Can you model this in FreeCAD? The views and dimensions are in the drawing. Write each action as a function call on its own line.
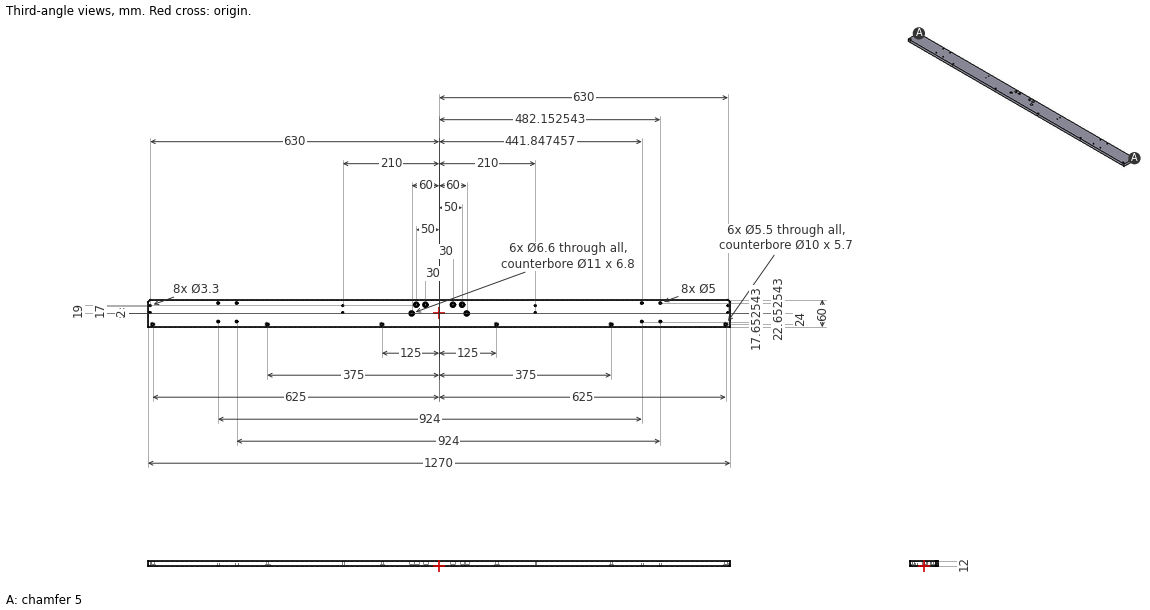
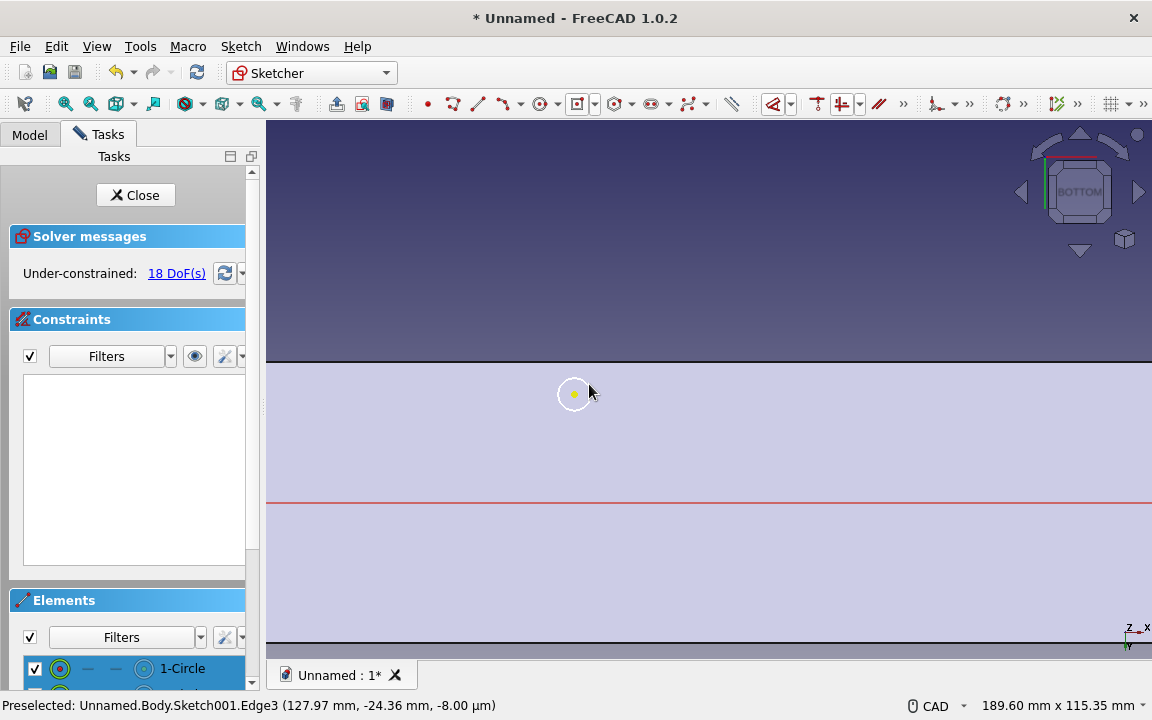
click(586, 383)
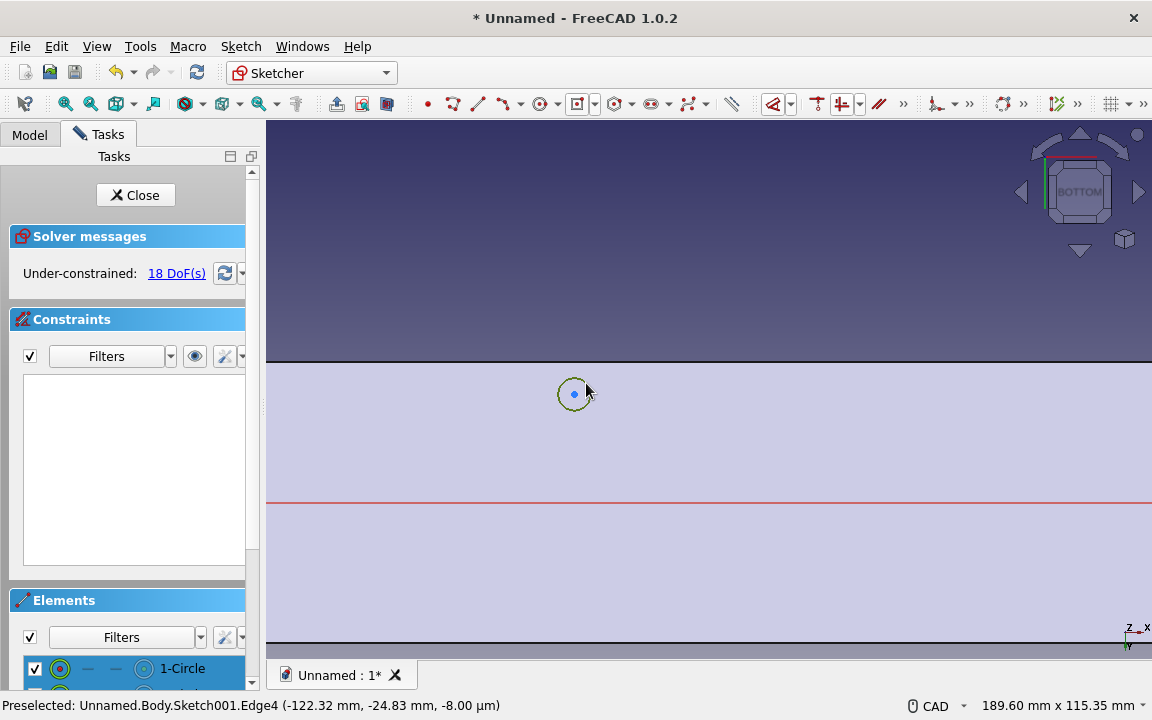
scroll(589, 384, down, 12)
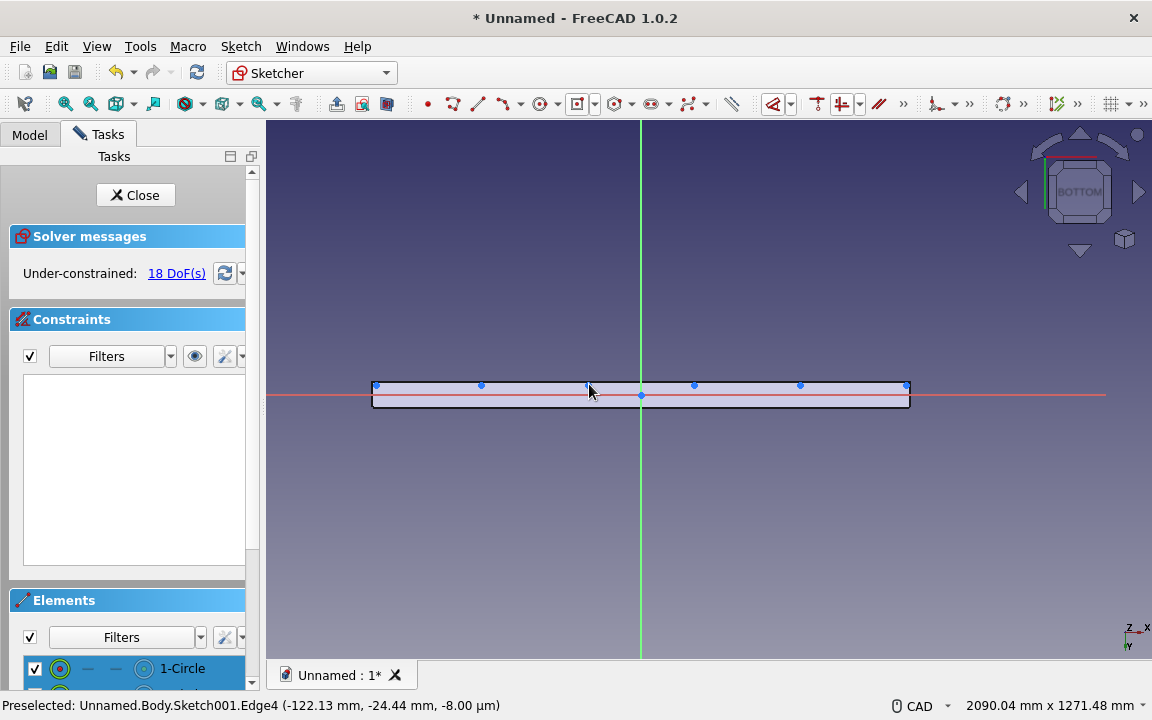
scroll(483, 384, up, 12)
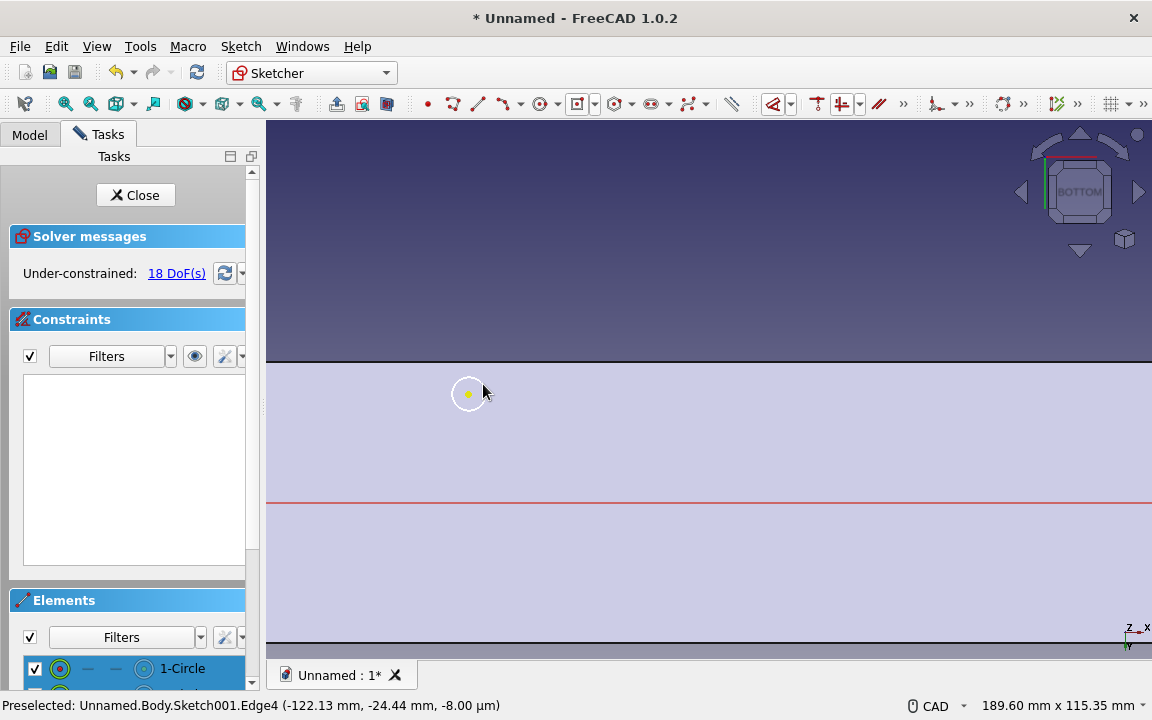
click(481, 382)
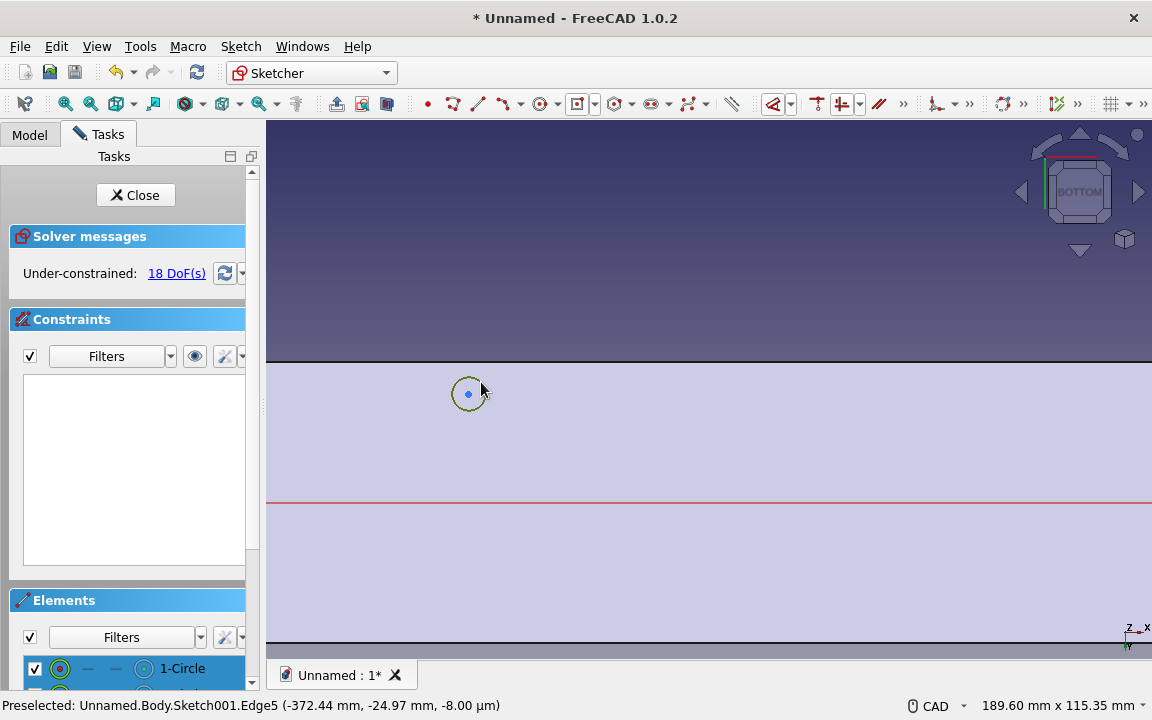
scroll(483, 384, down, 12)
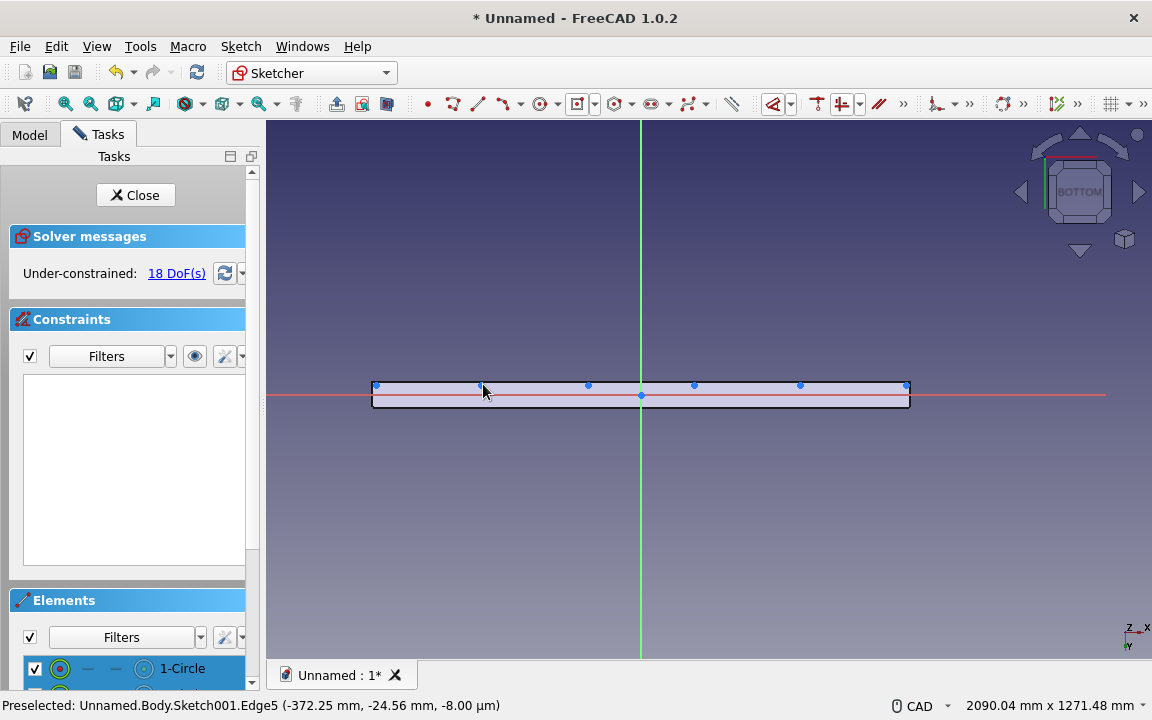
scroll(378, 385, up, 11)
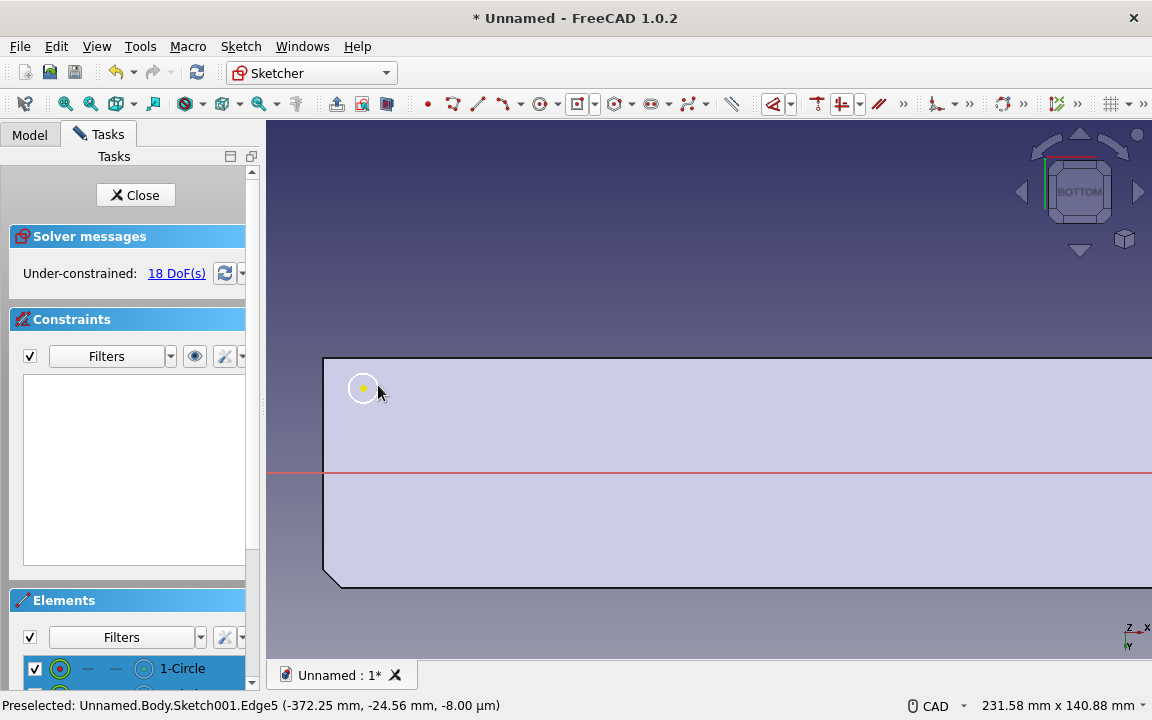
click(374, 378)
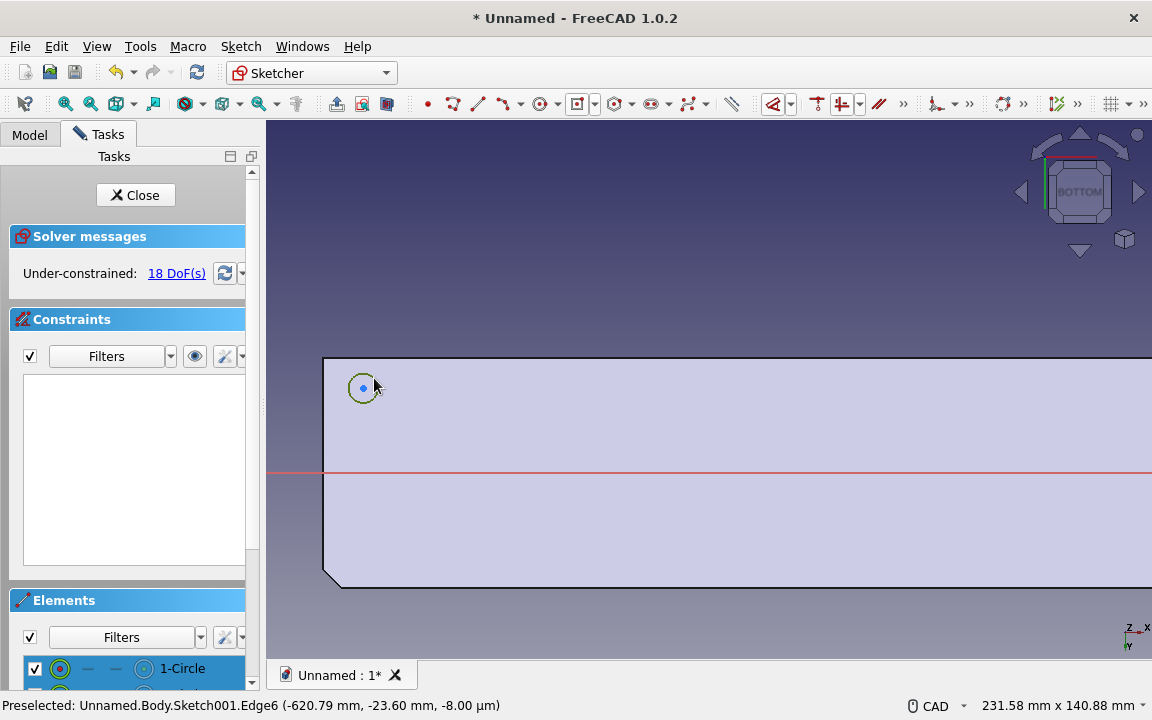
key(e)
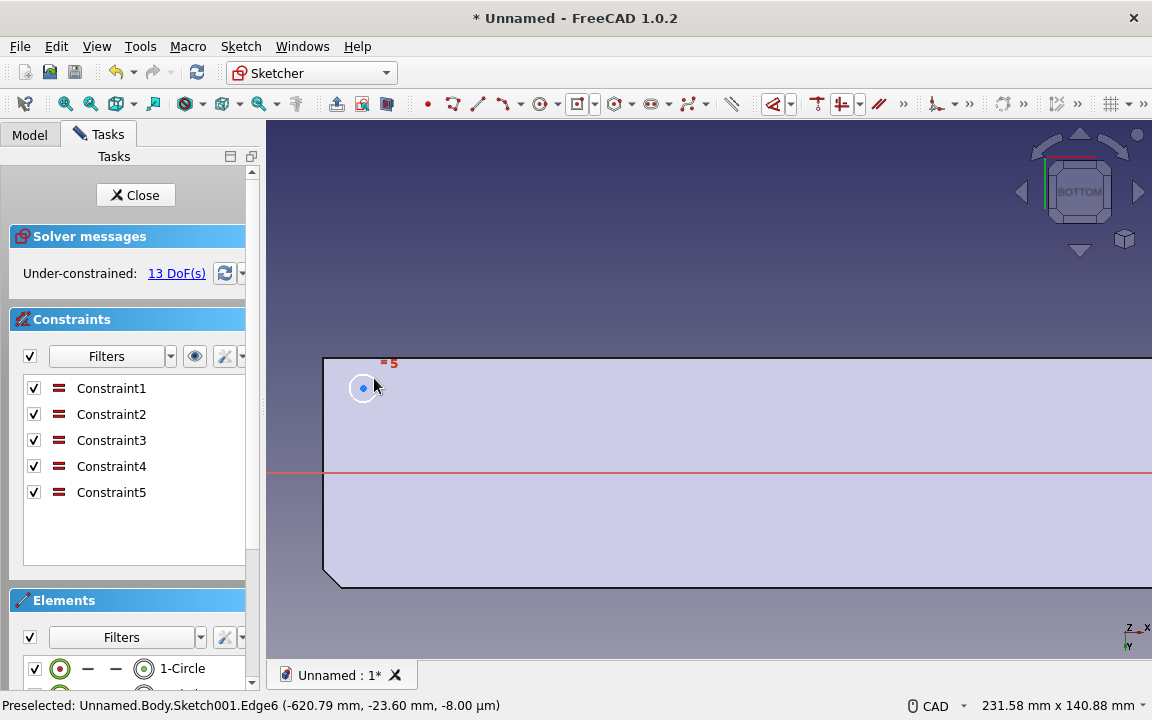
scroll(377, 385, down, 11)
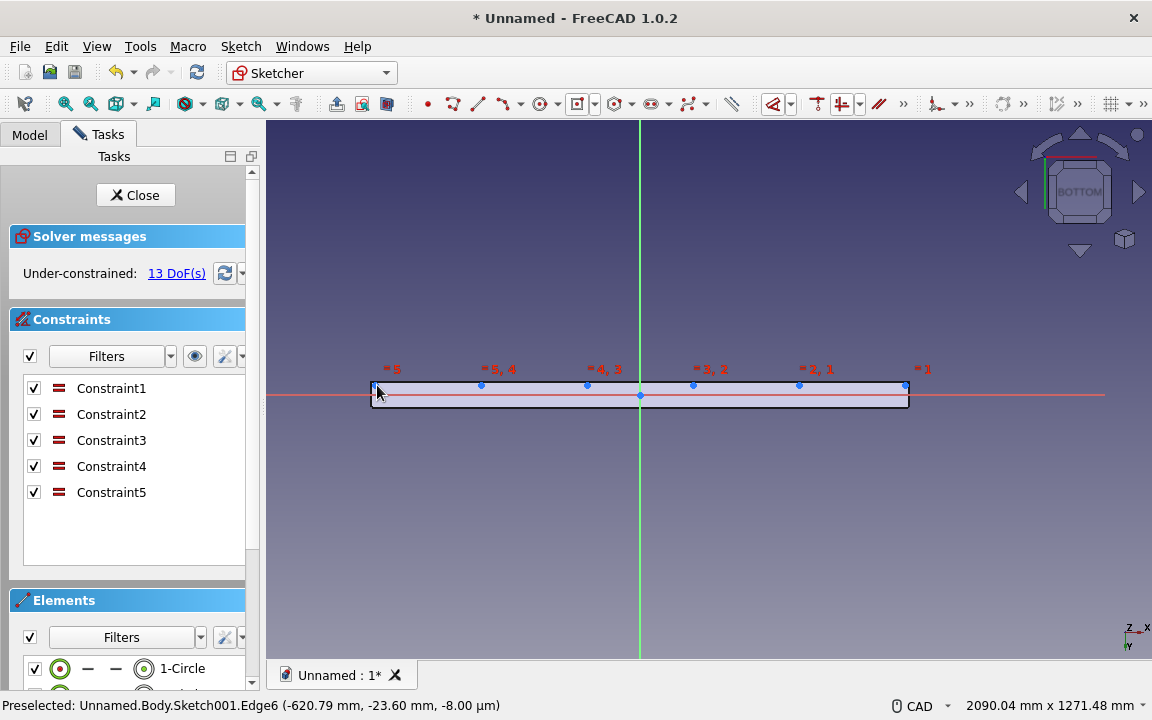
click(905, 386)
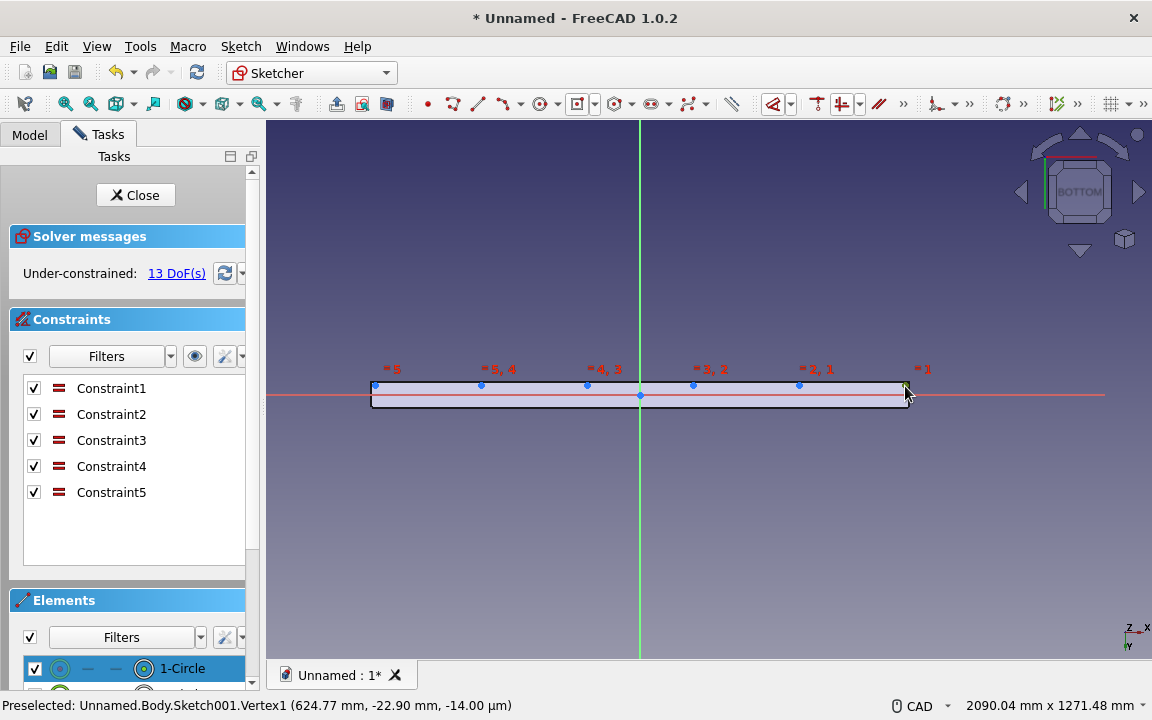
click(799, 385)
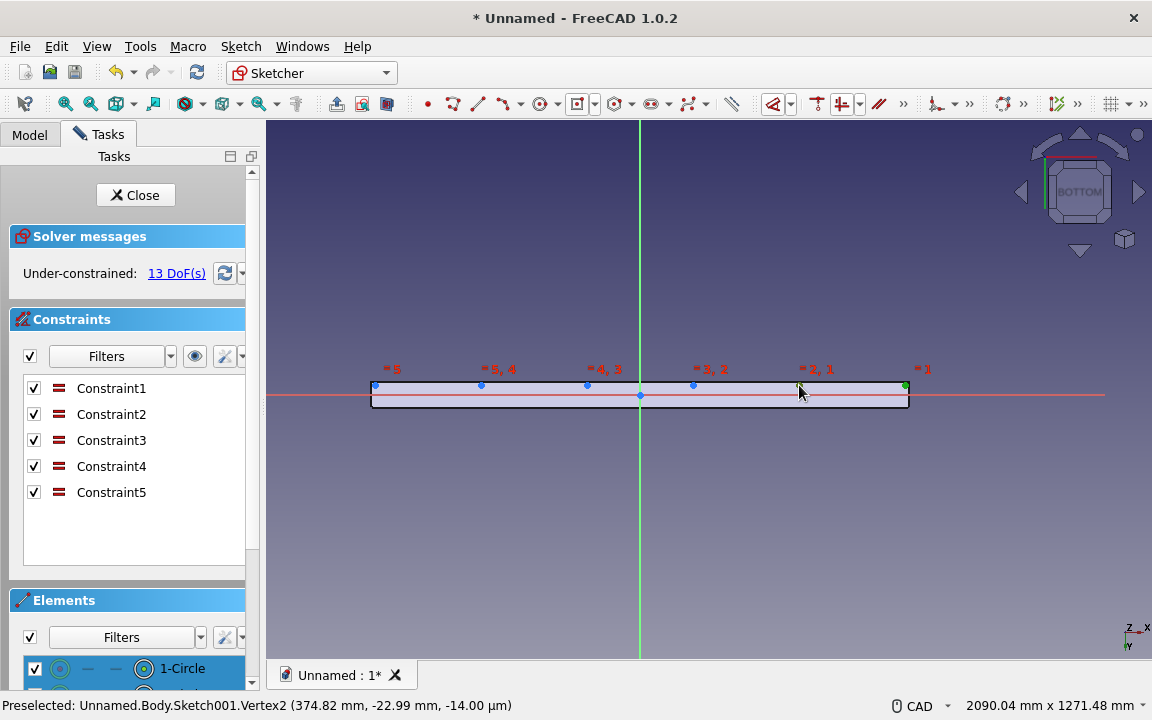
key(h)